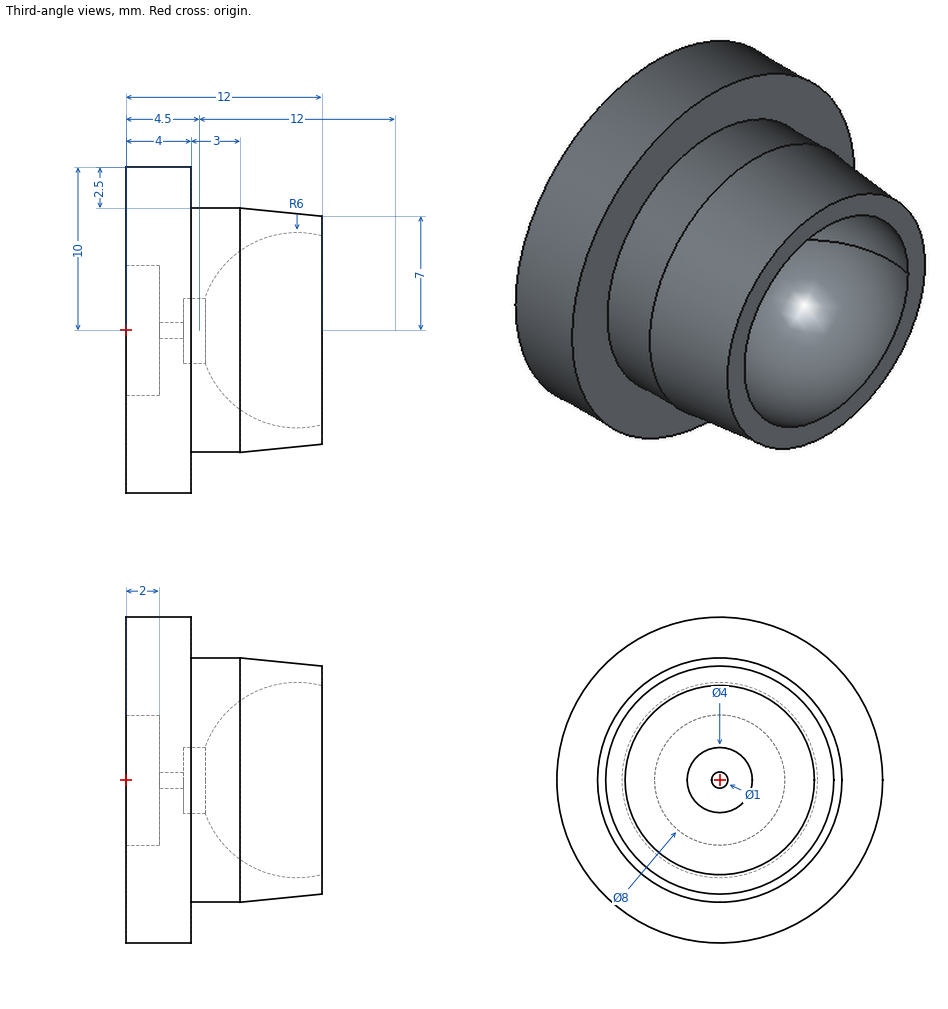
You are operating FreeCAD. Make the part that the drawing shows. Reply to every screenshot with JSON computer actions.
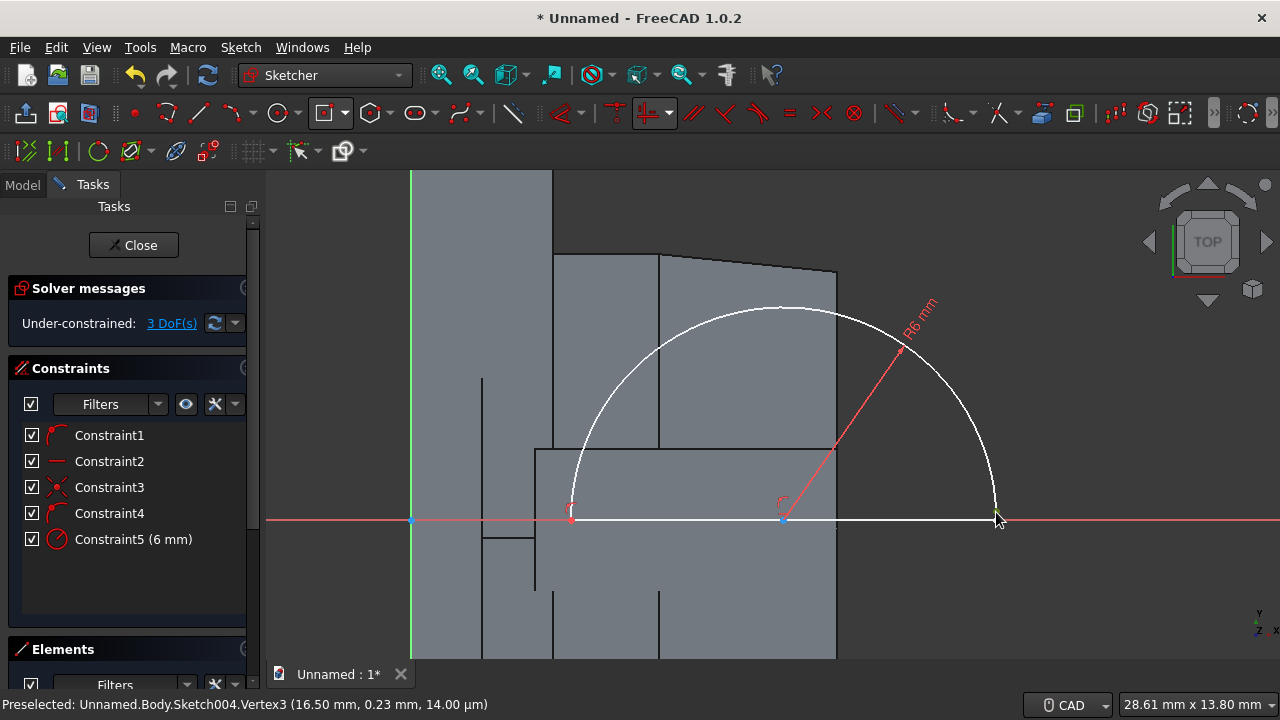
{"action": "left_click", "coordinate": [353, 520]}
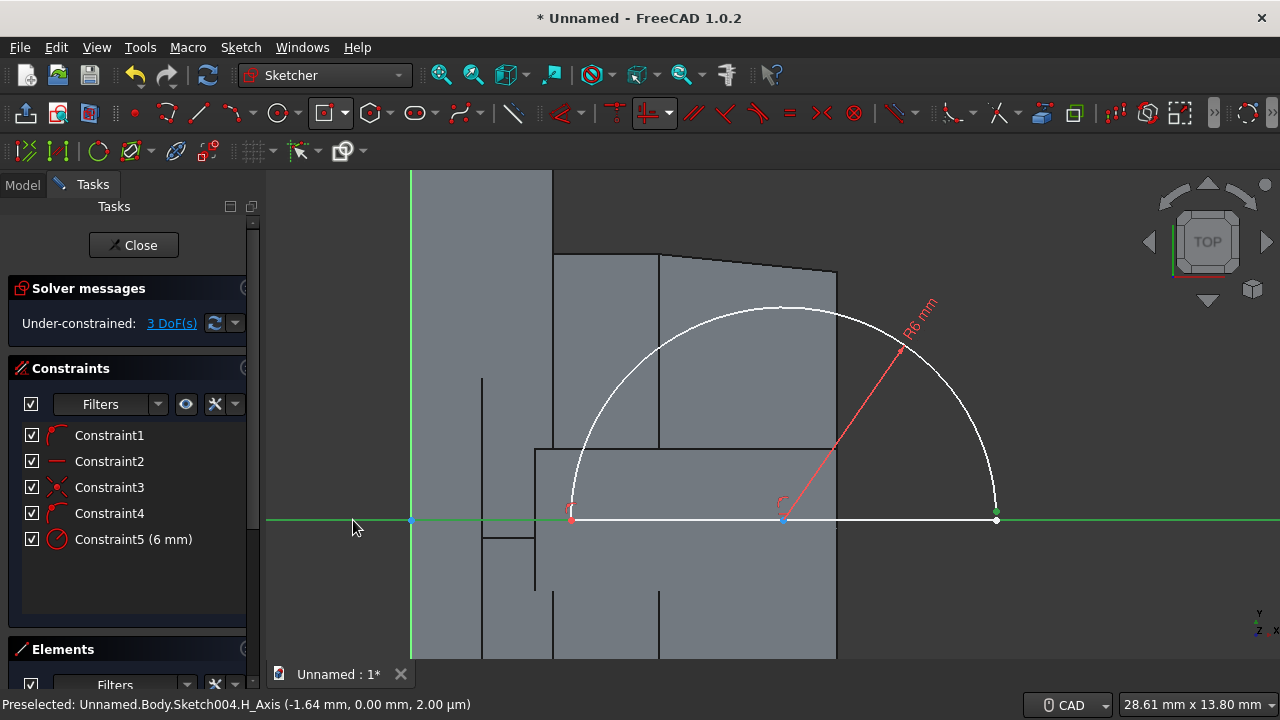
{"action": "left_click", "coordinate": [616, 114]}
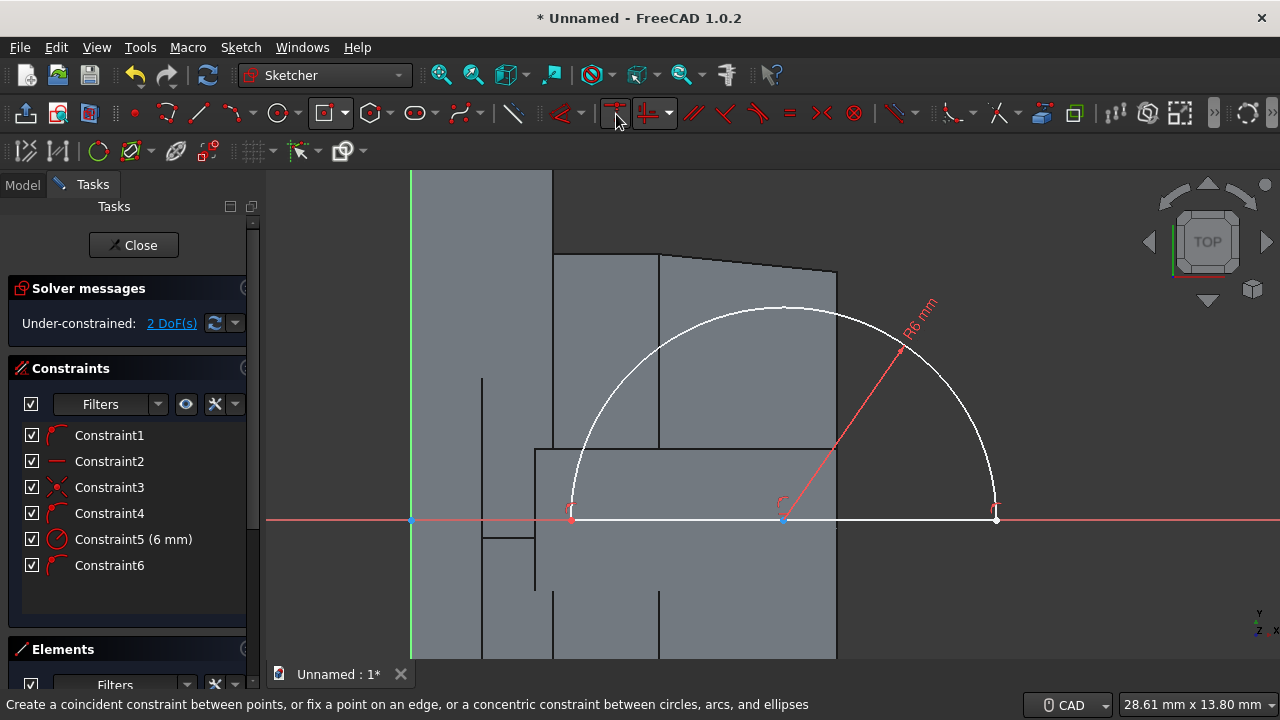
{"action": "left_click", "coordinate": [560, 114]}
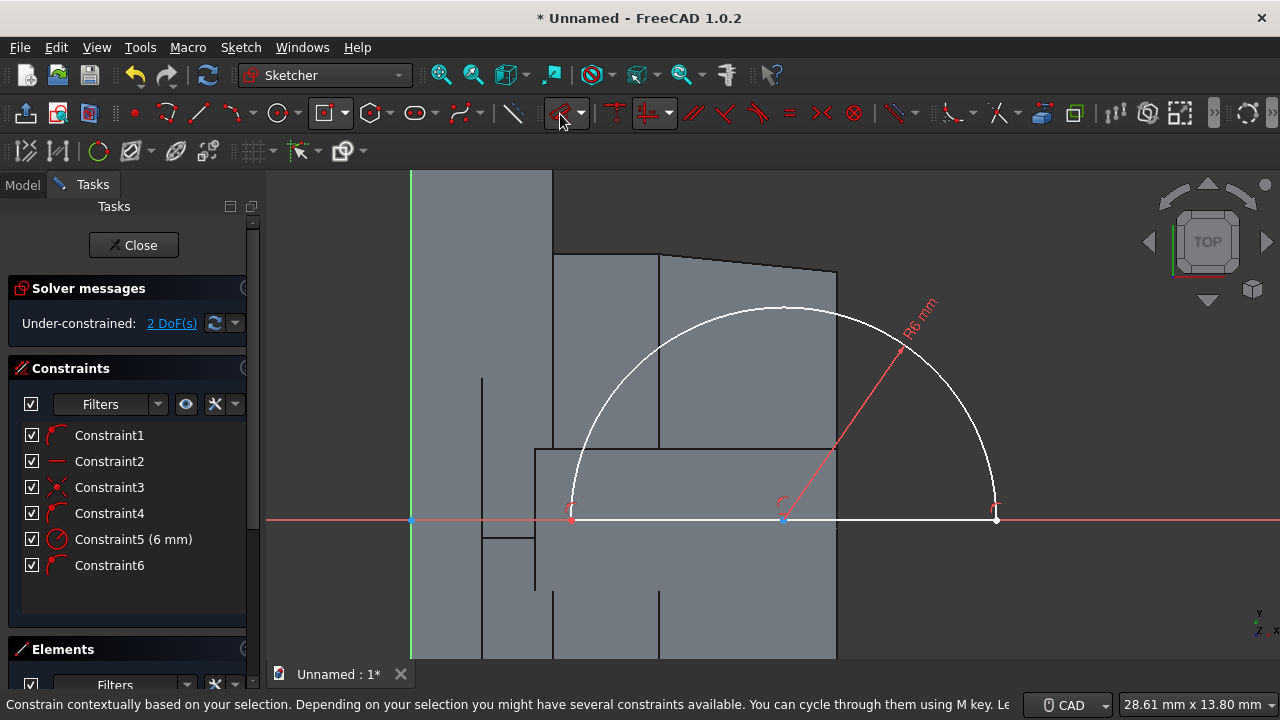
{"action": "left_click", "coordinate": [699, 520]}
{"action": "left_click", "coordinate": [784, 554]}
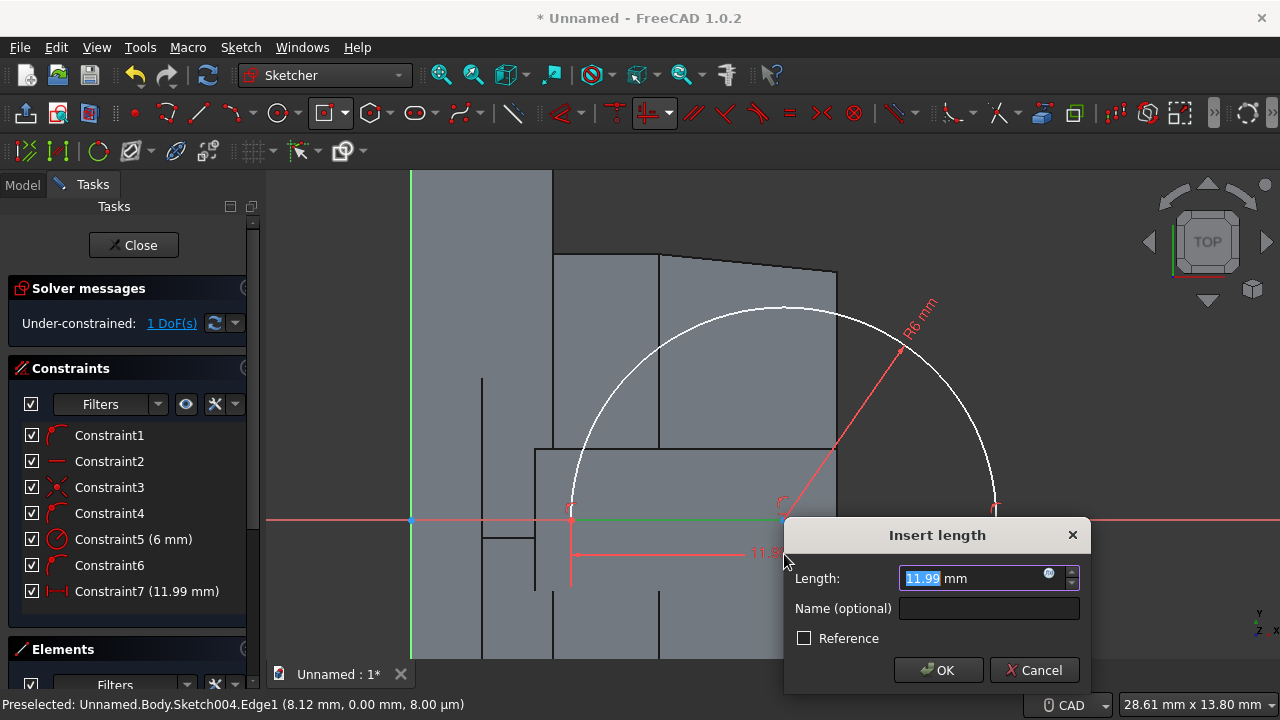
{"action": "type", "text": "12"}
{"action": "key", "text": "Return"}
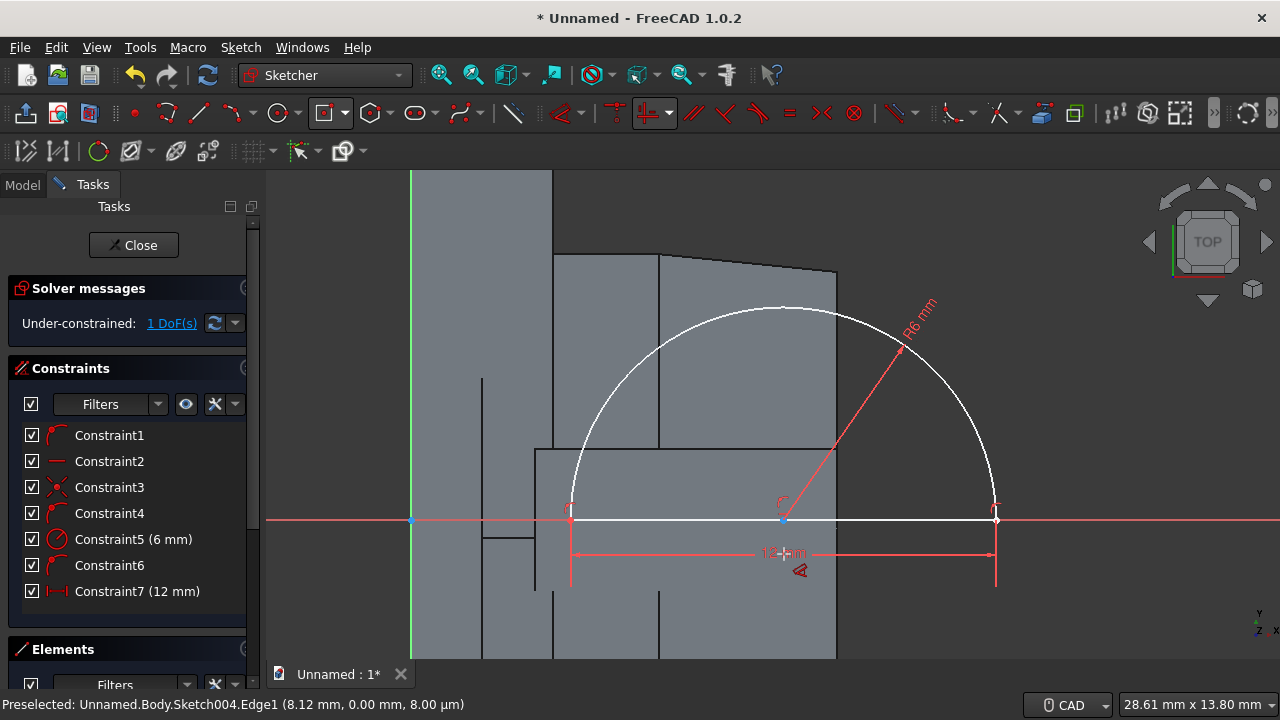
{"action": "left_click", "coordinate": [571, 520]}
{"action": "left_click", "coordinate": [491, 554]}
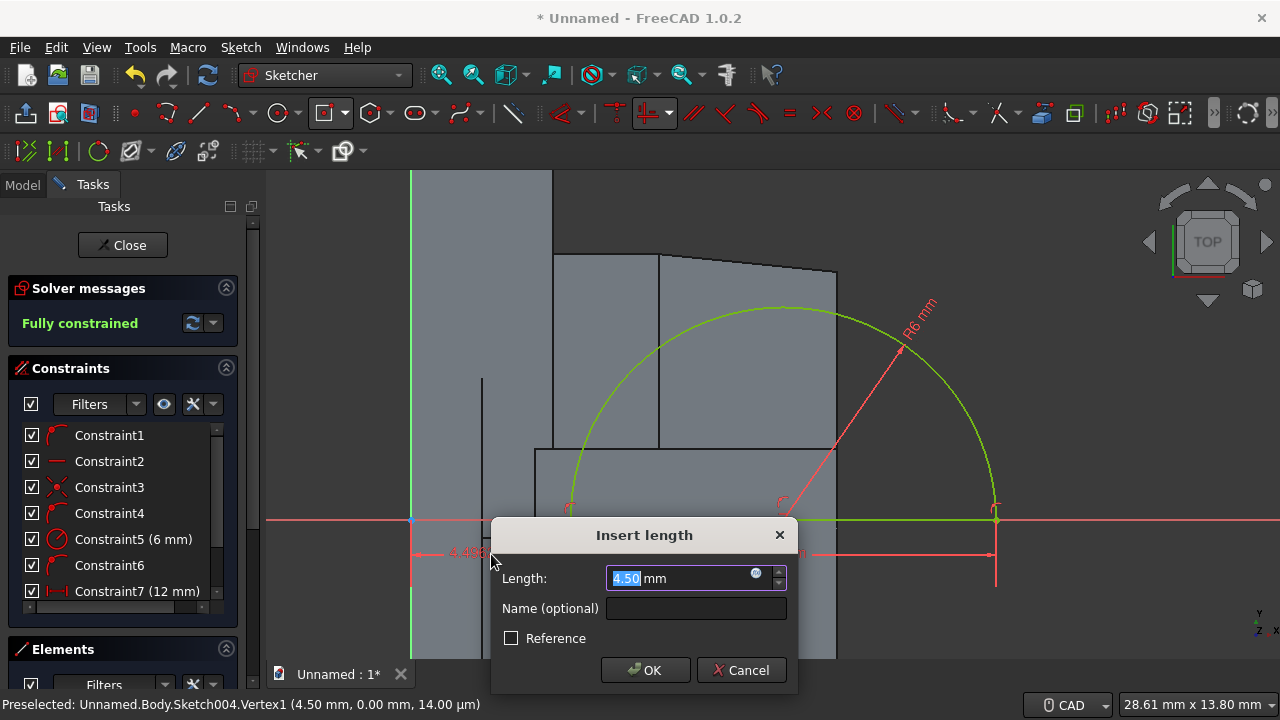
{"action": "type", "text": "4.5"}
{"action": "key", "text": "Return"}
{"action": "key", "text": "Escape"}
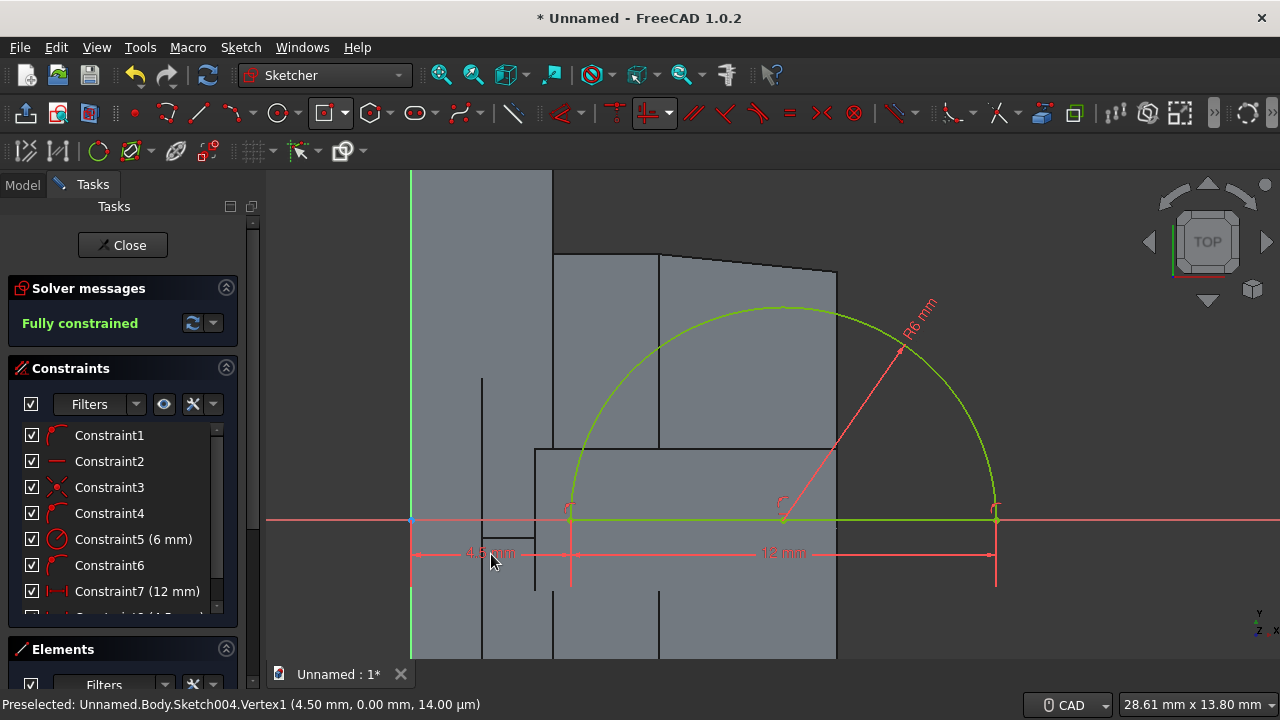
{"action": "left_click", "coordinate": [123, 245]}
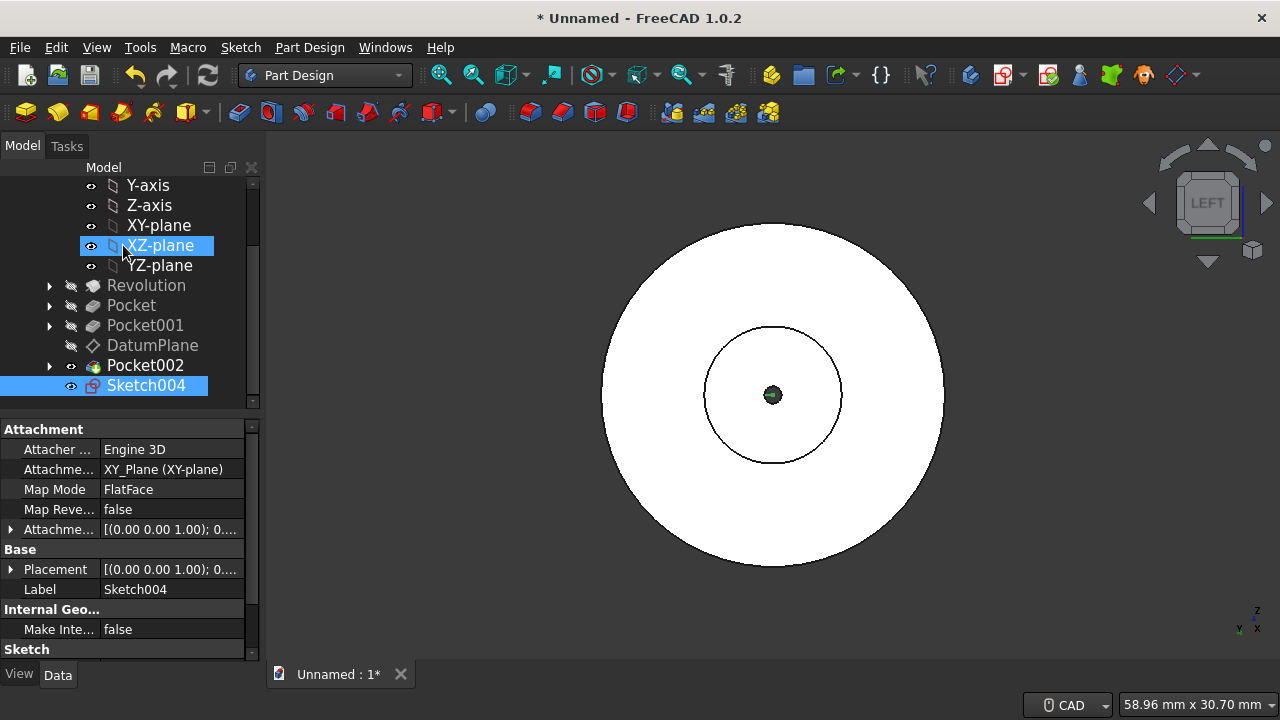
{"action": "left_click", "coordinate": [304, 112]}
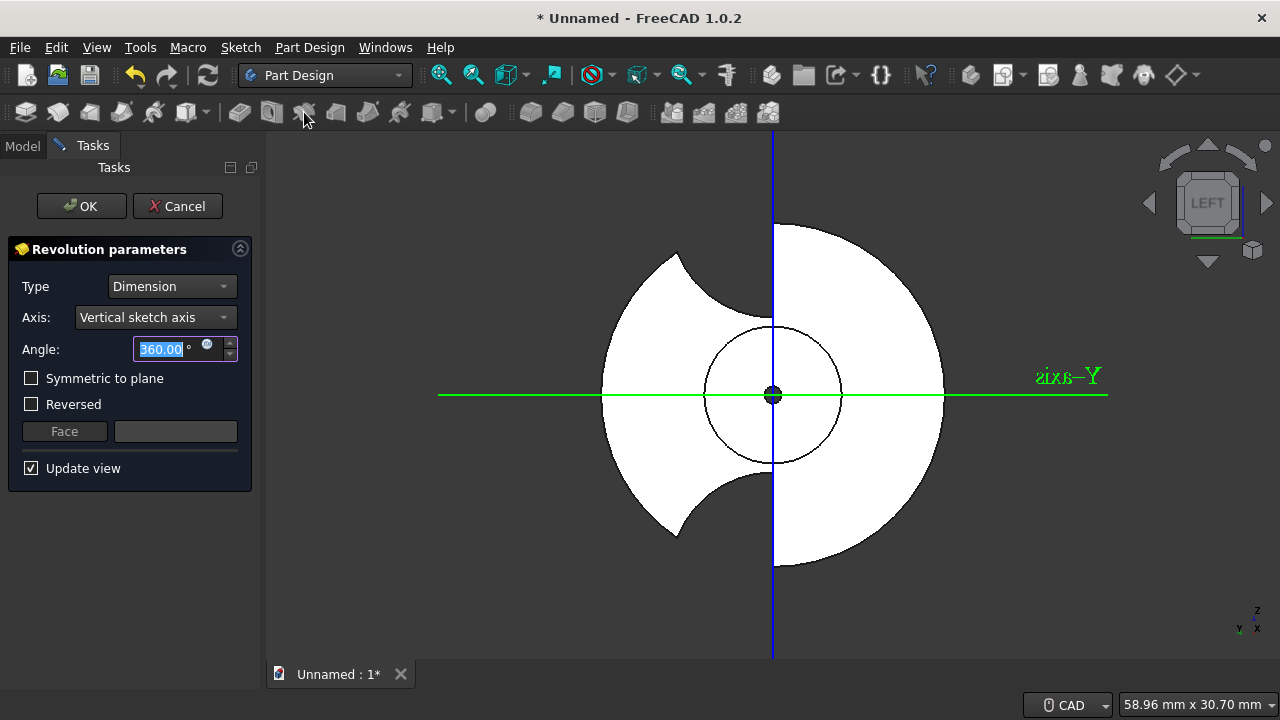
{"action": "left_click", "coordinate": [156, 318]}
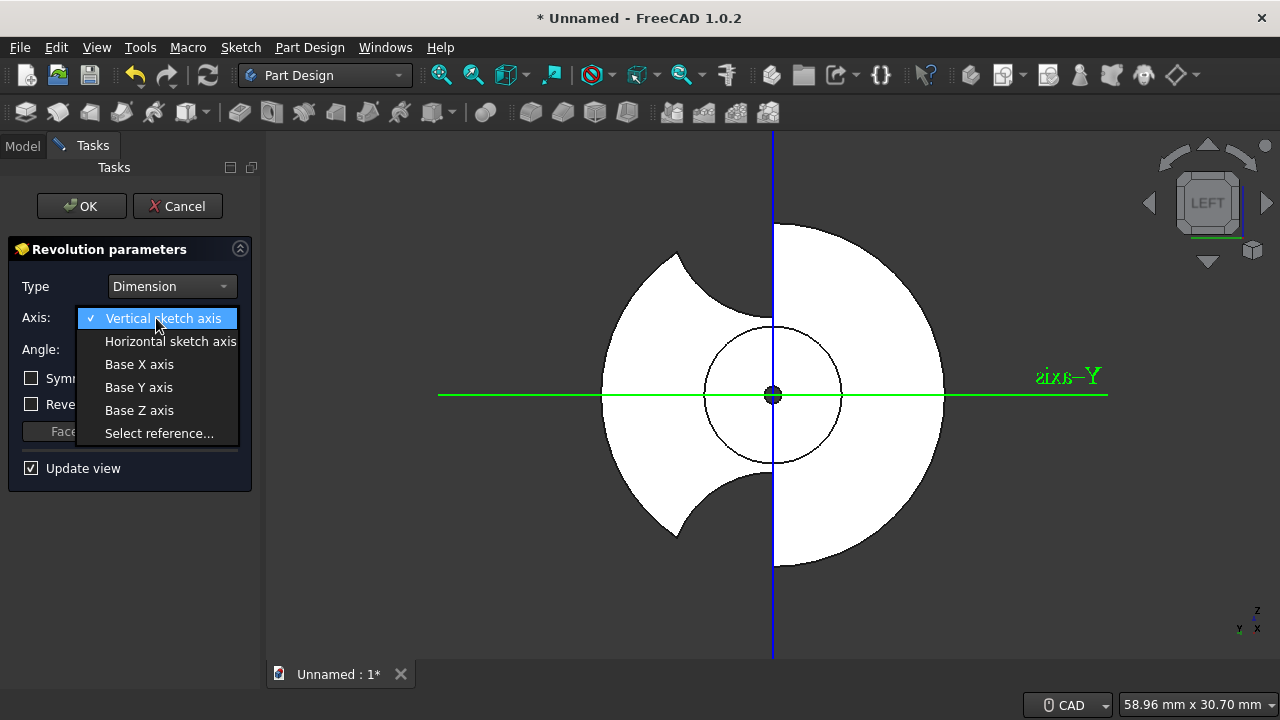
{"action": "left_click", "coordinate": [156, 342]}